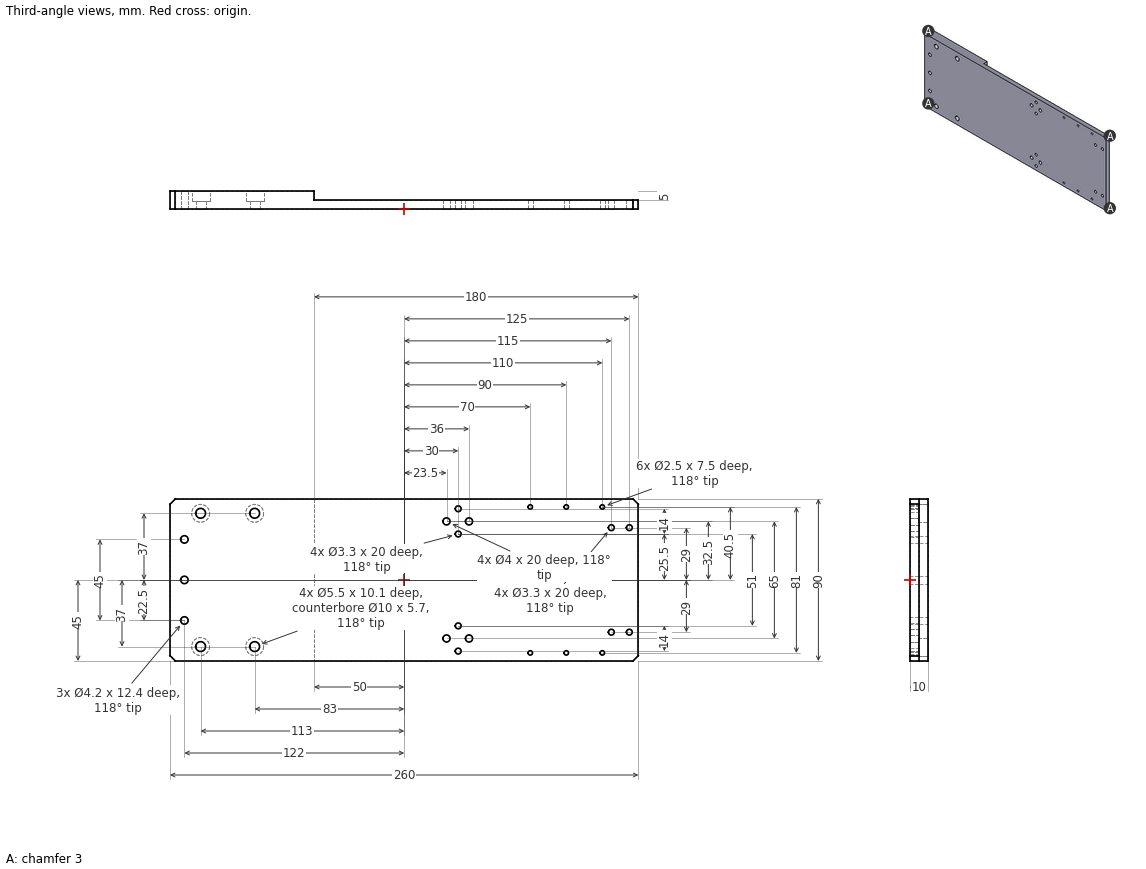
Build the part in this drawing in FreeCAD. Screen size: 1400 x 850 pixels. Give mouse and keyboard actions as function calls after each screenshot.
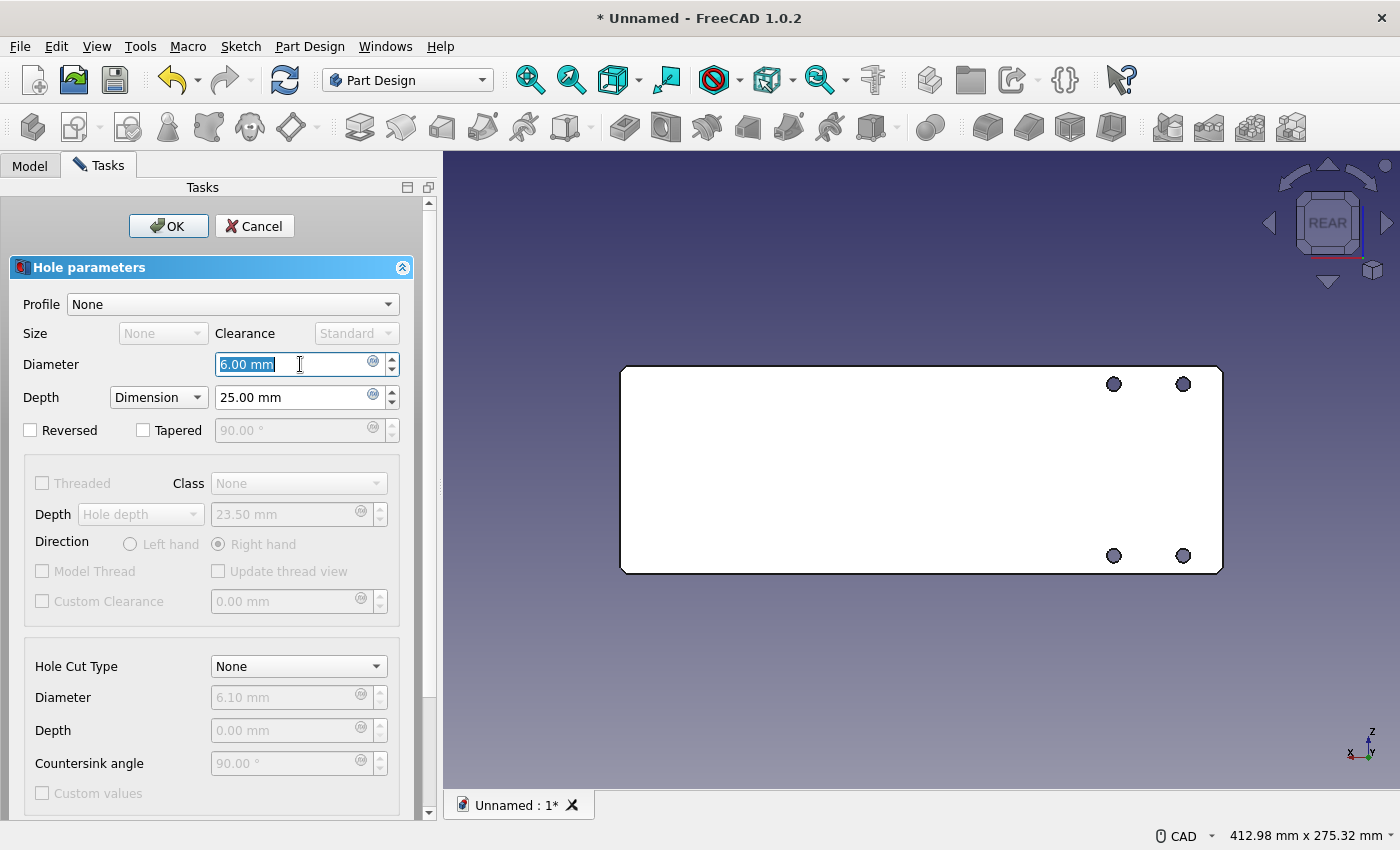
text(5.5)
key(Tab)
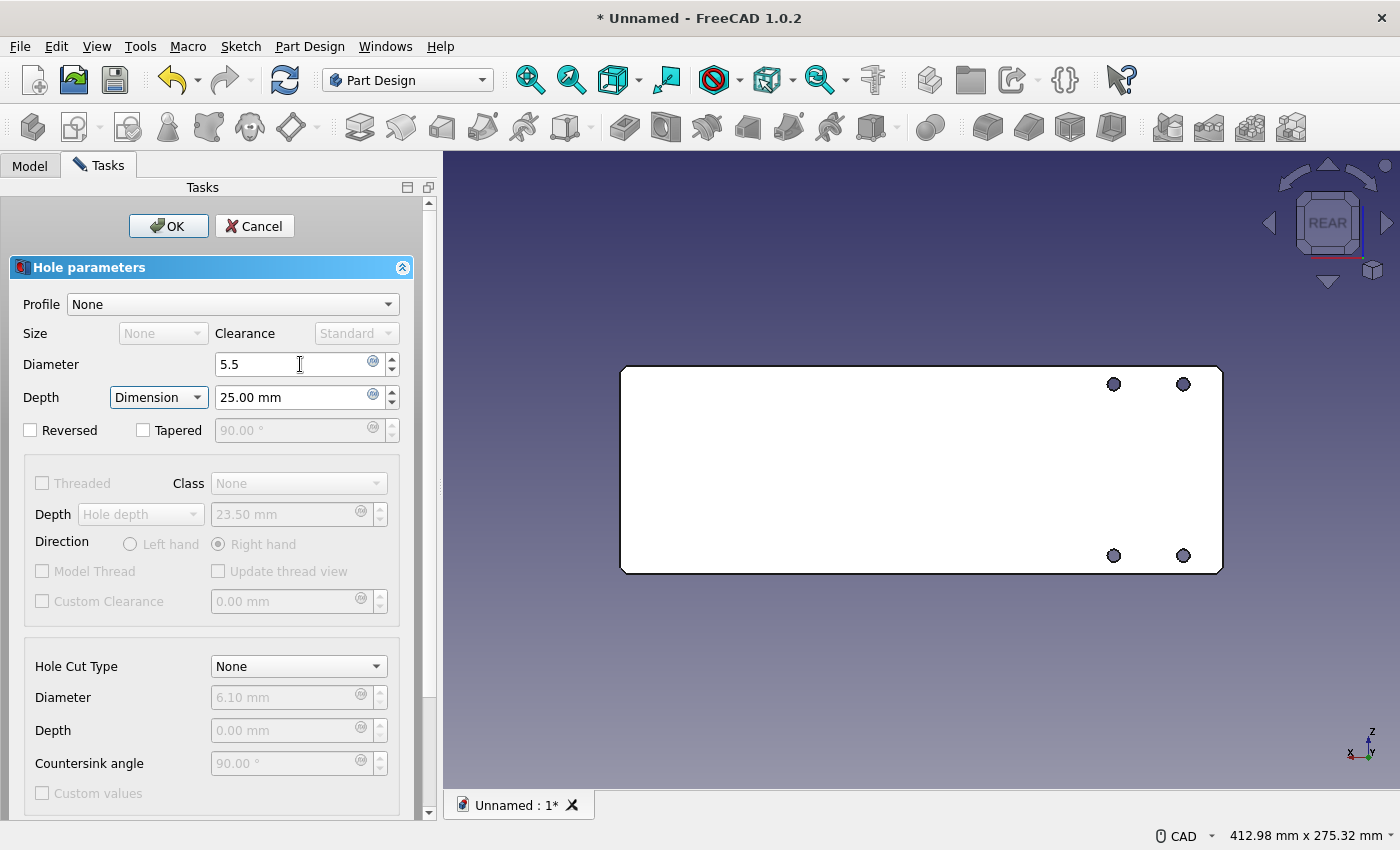
triple_click(300, 398)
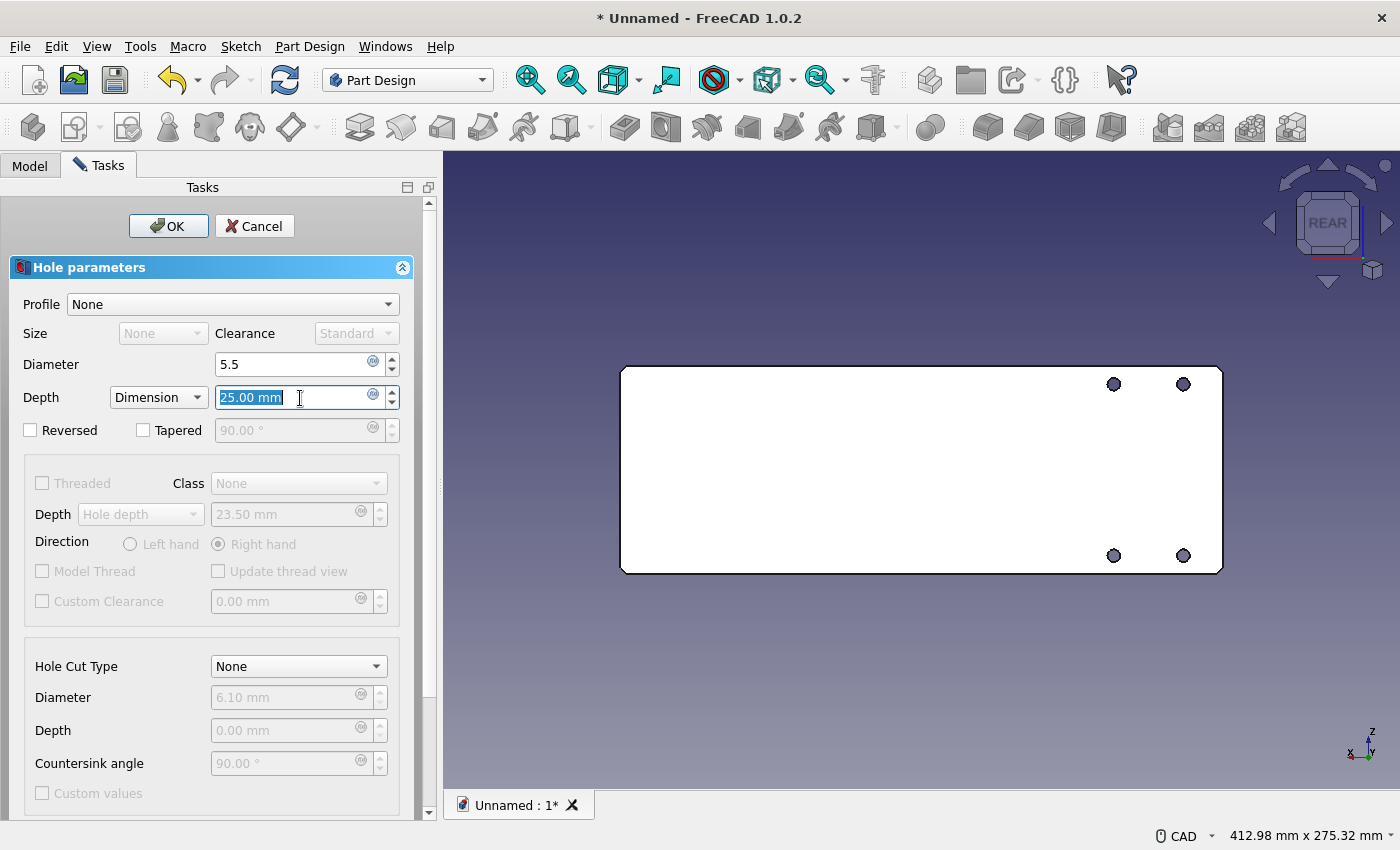
text(10.1)
key(Tab)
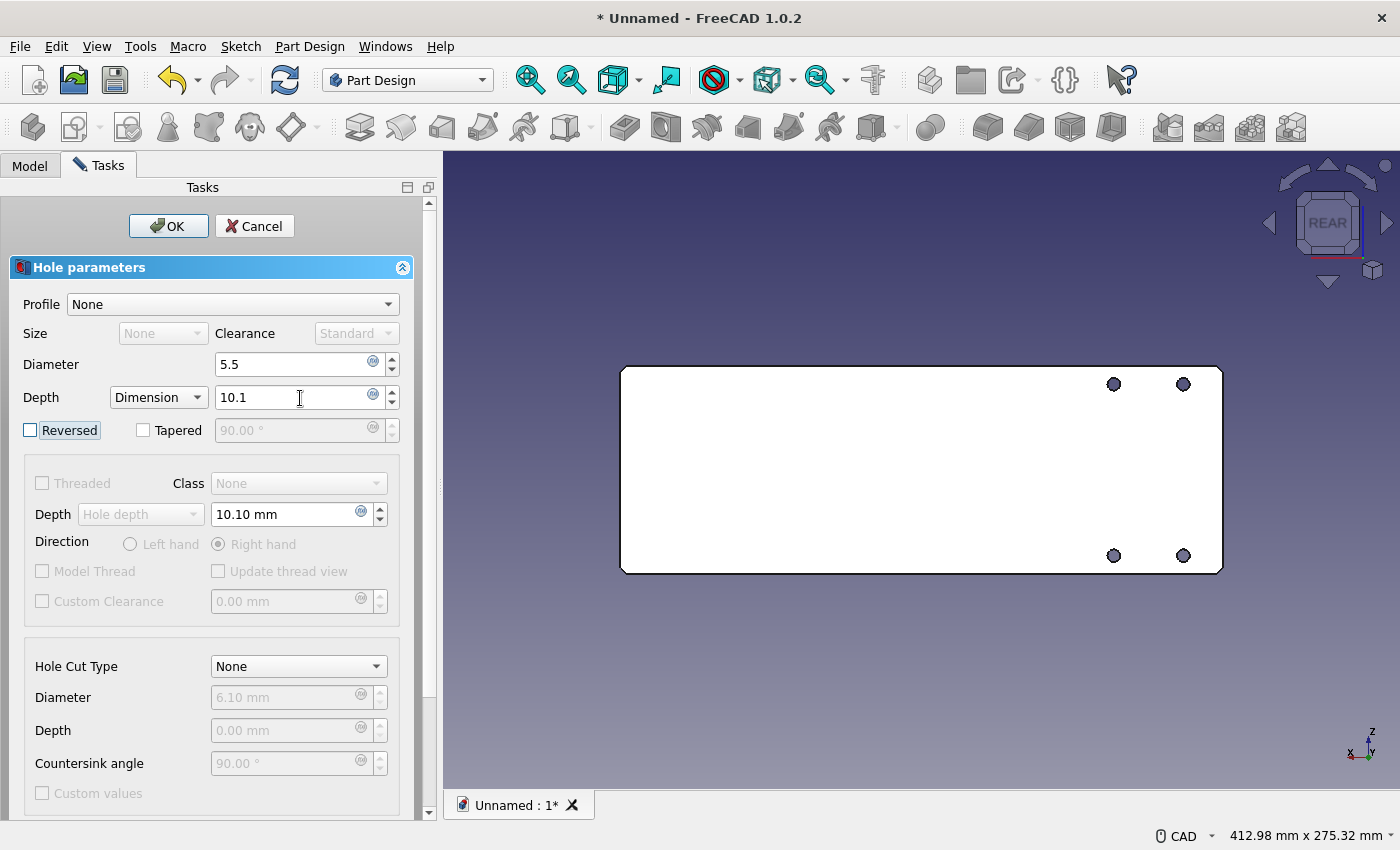
click(300, 666)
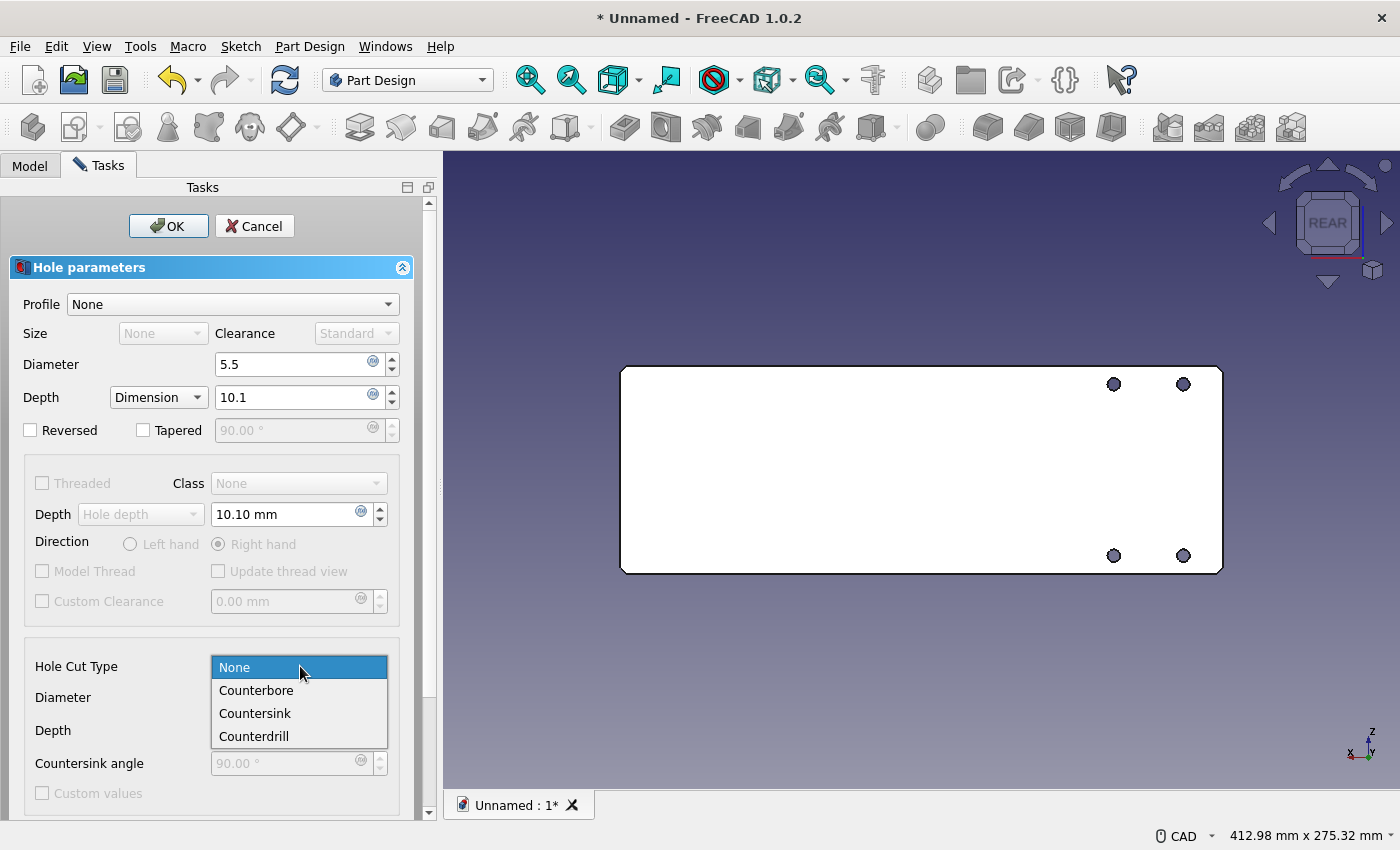
click(298, 690)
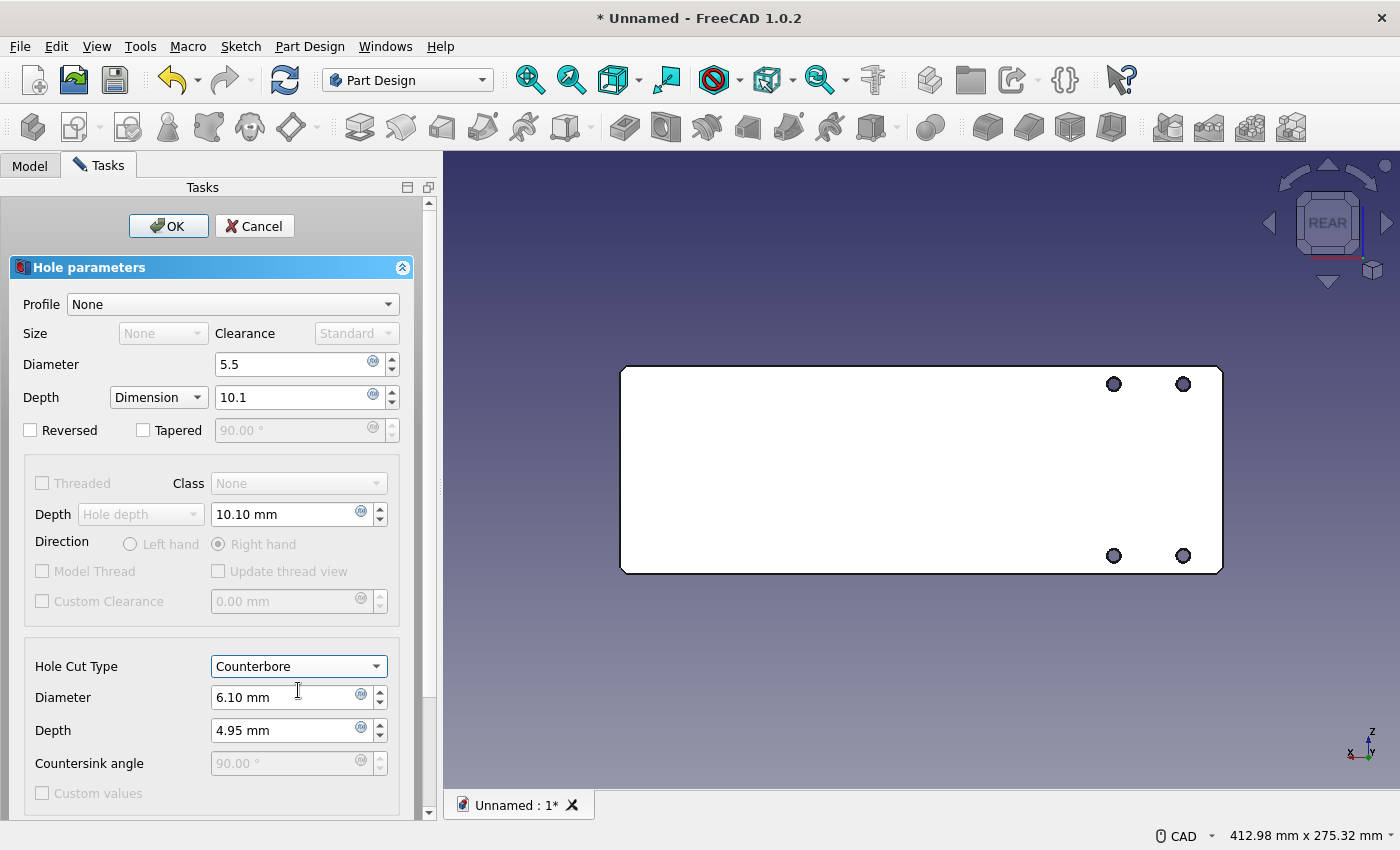
triple_click(292, 698)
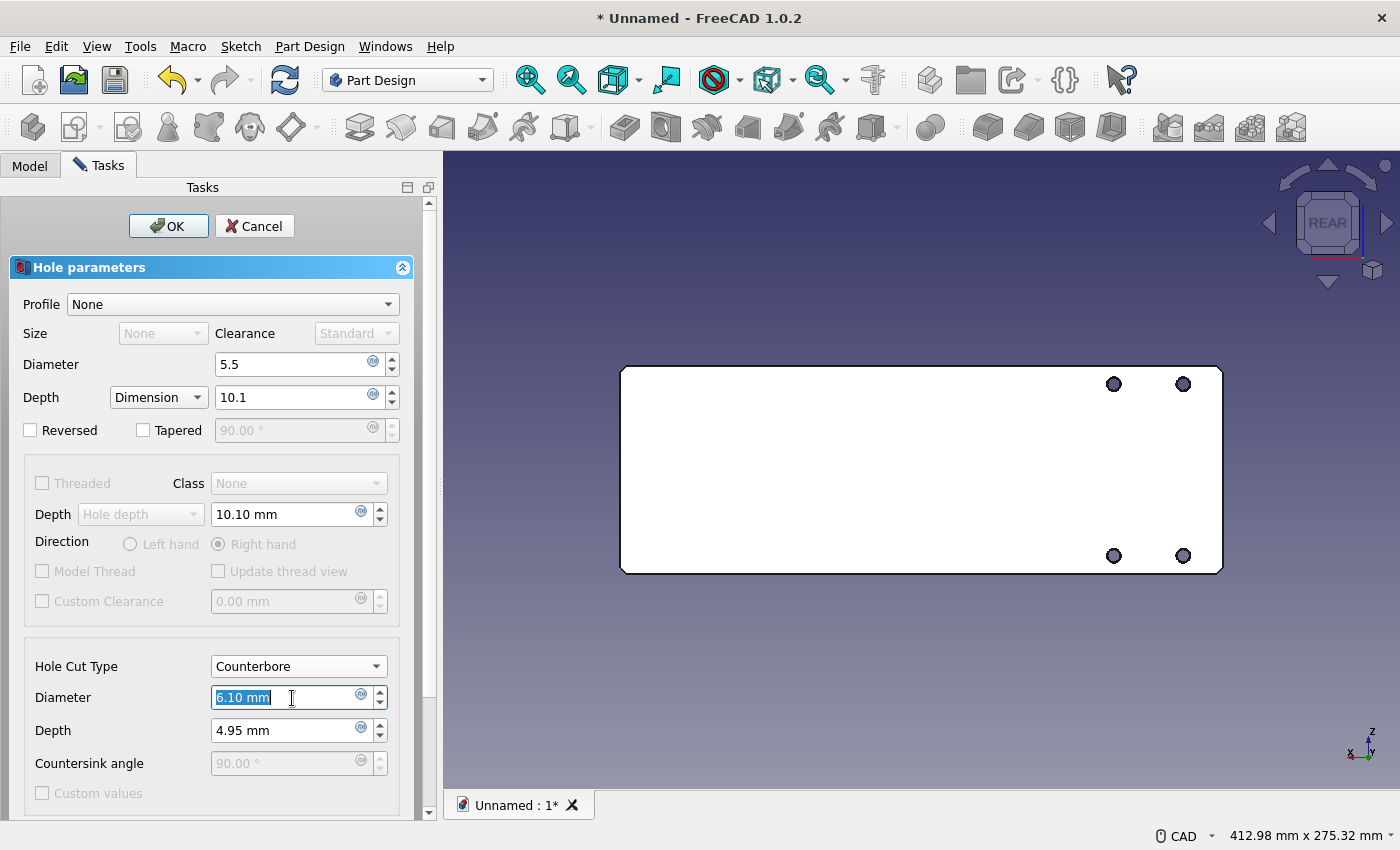
text(10)
key(Tab)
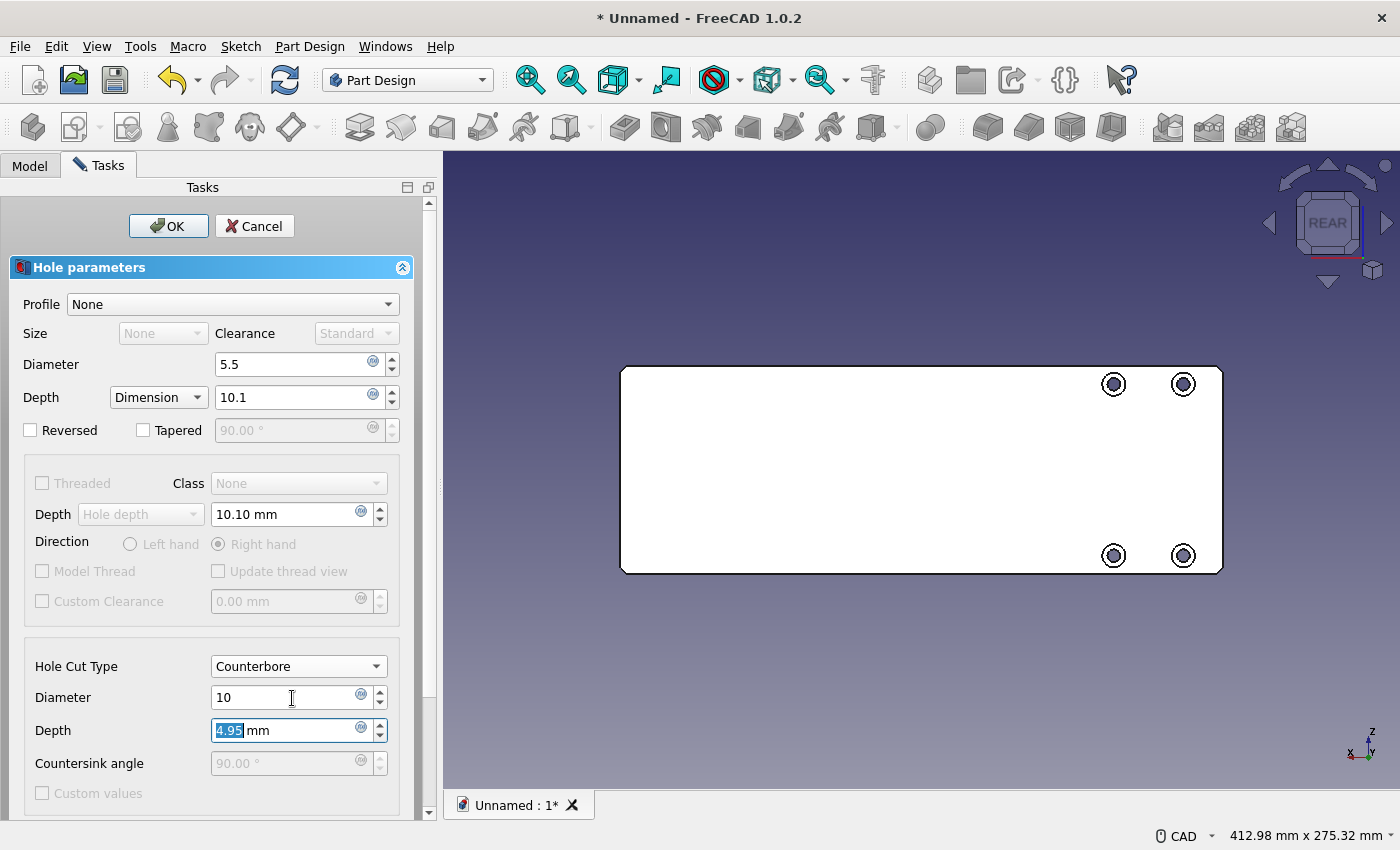
text(5.7)
key(Tab)